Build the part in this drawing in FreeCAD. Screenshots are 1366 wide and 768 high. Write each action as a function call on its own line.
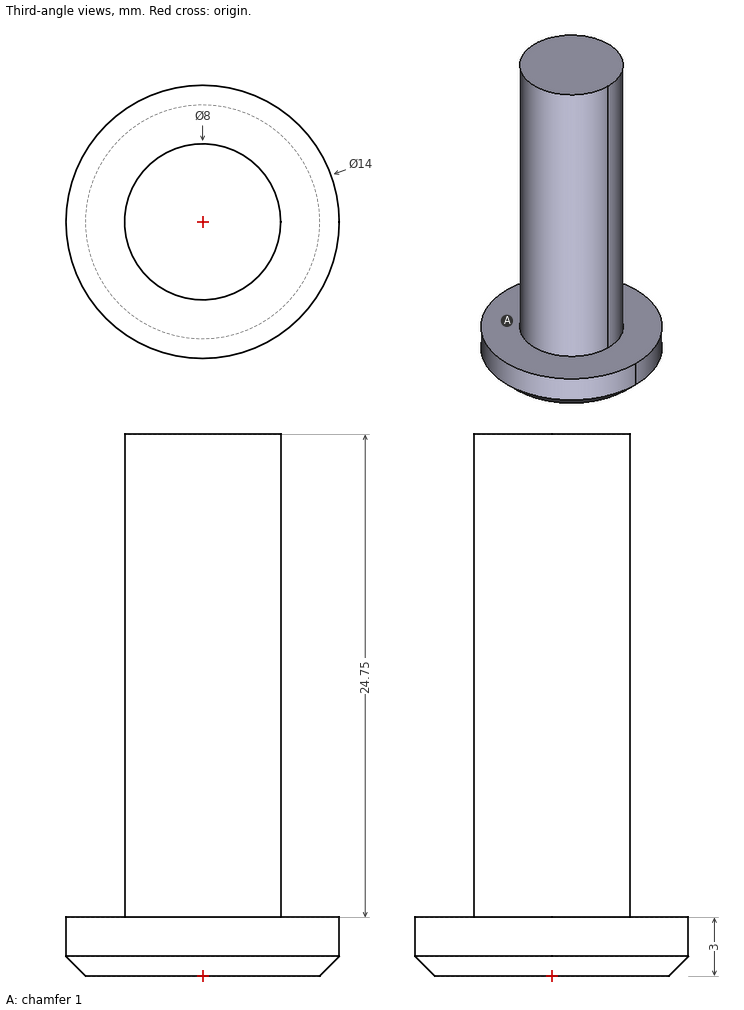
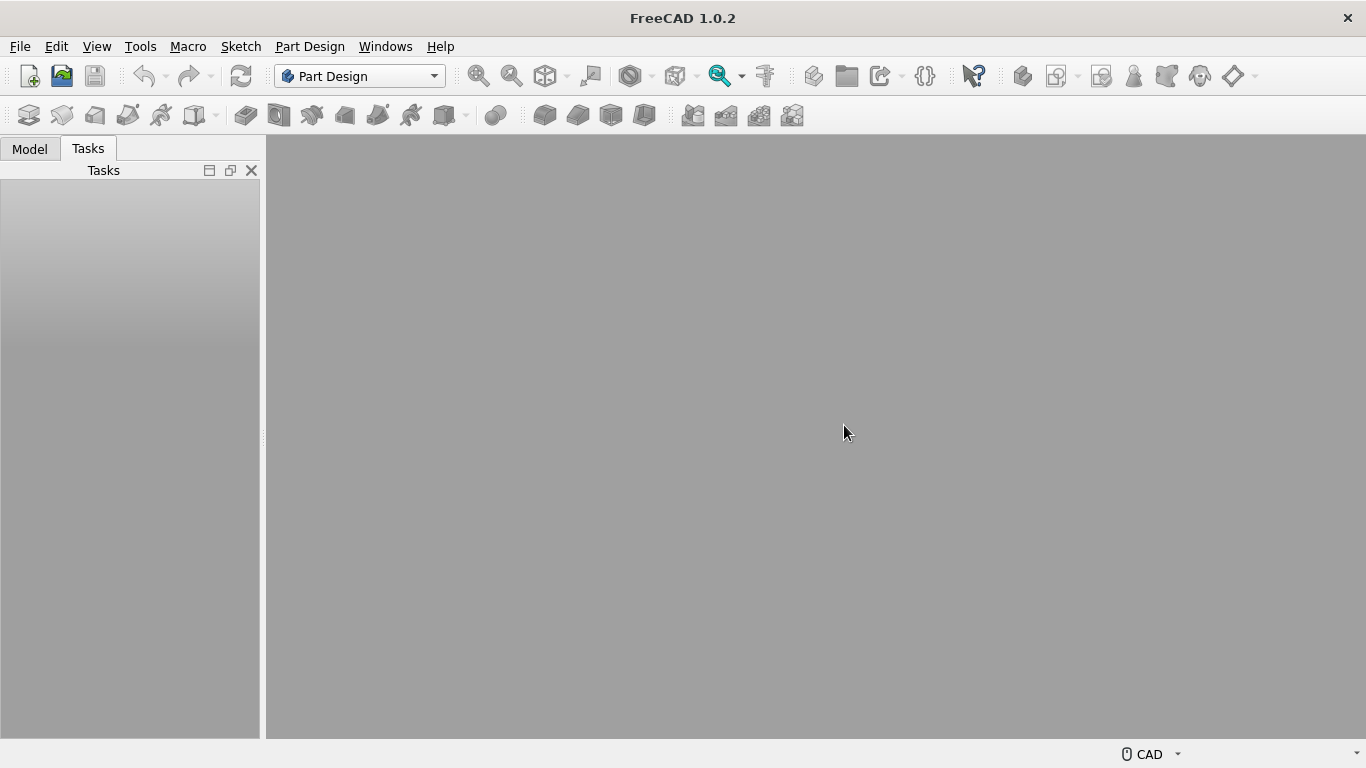
click(29, 76)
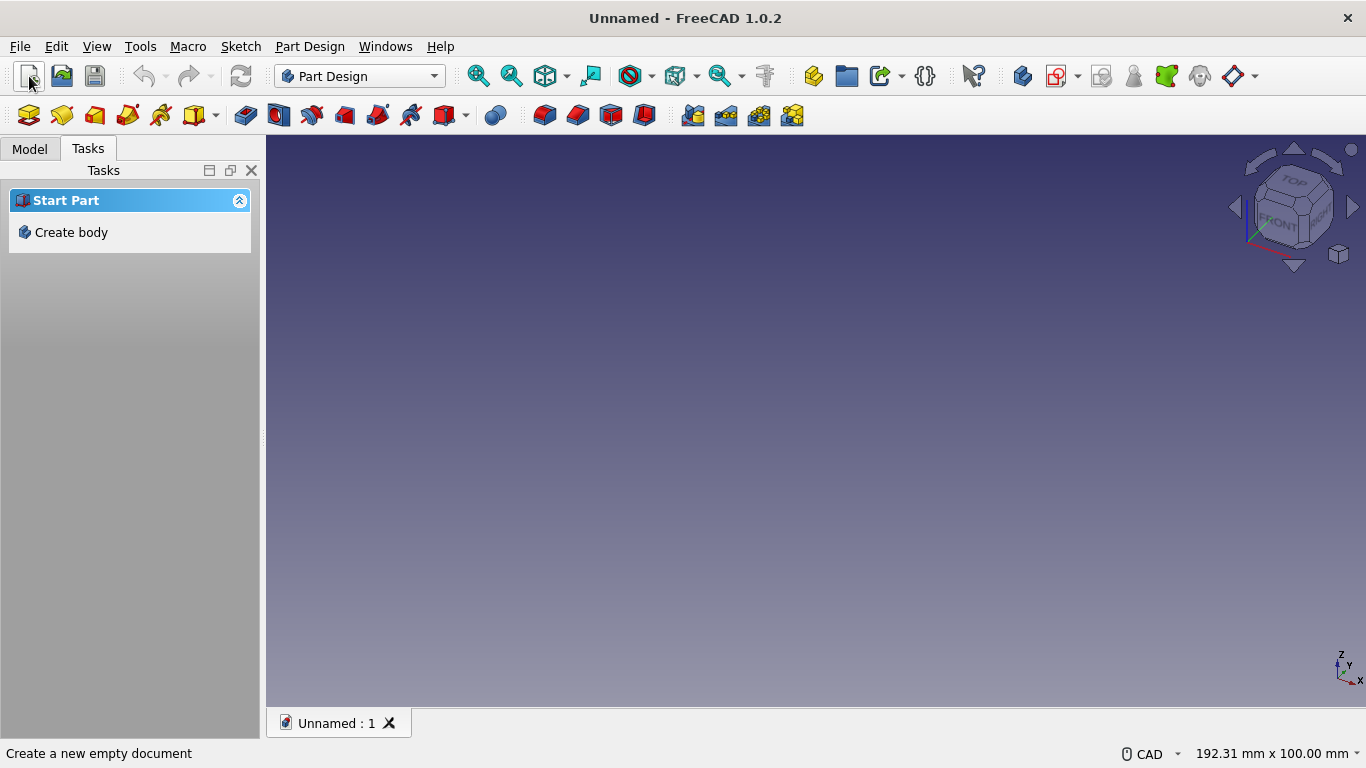
click(1056, 76)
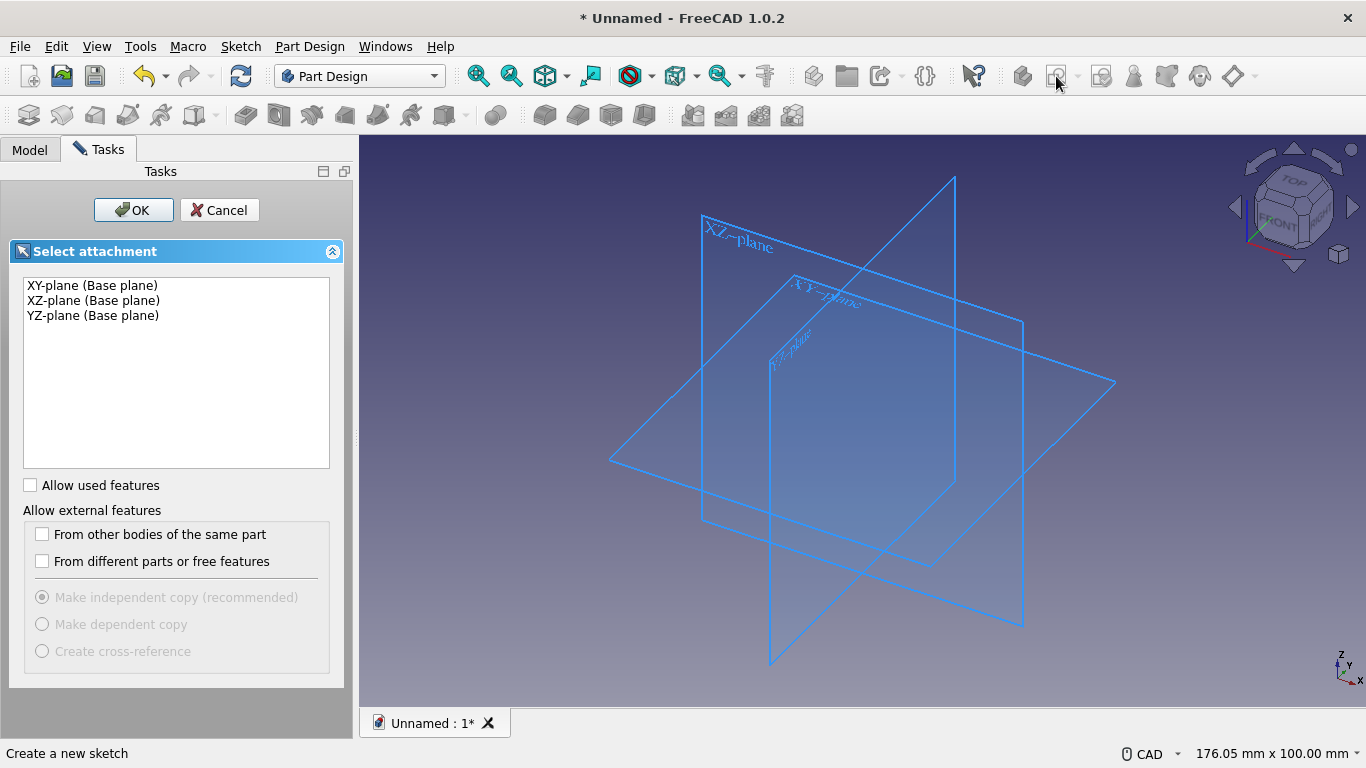
click(84, 286)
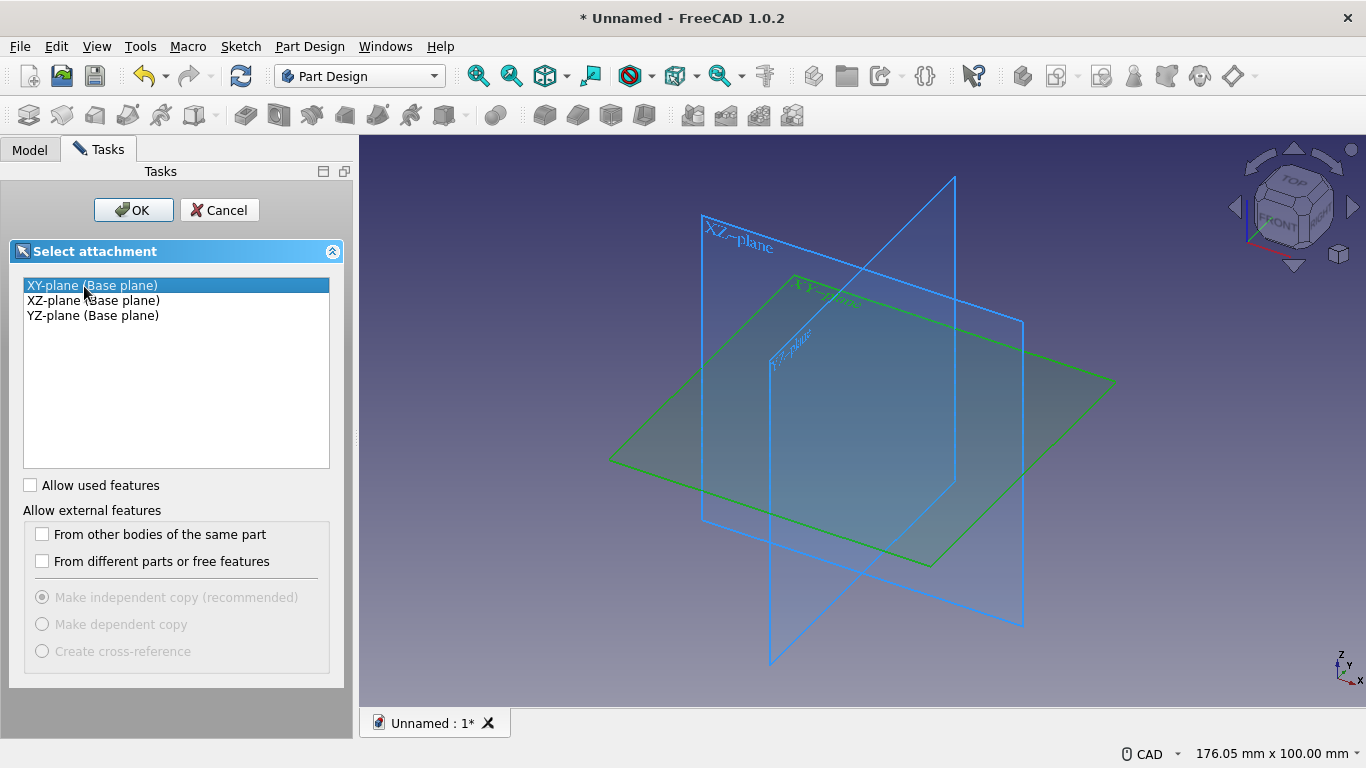
click(134, 210)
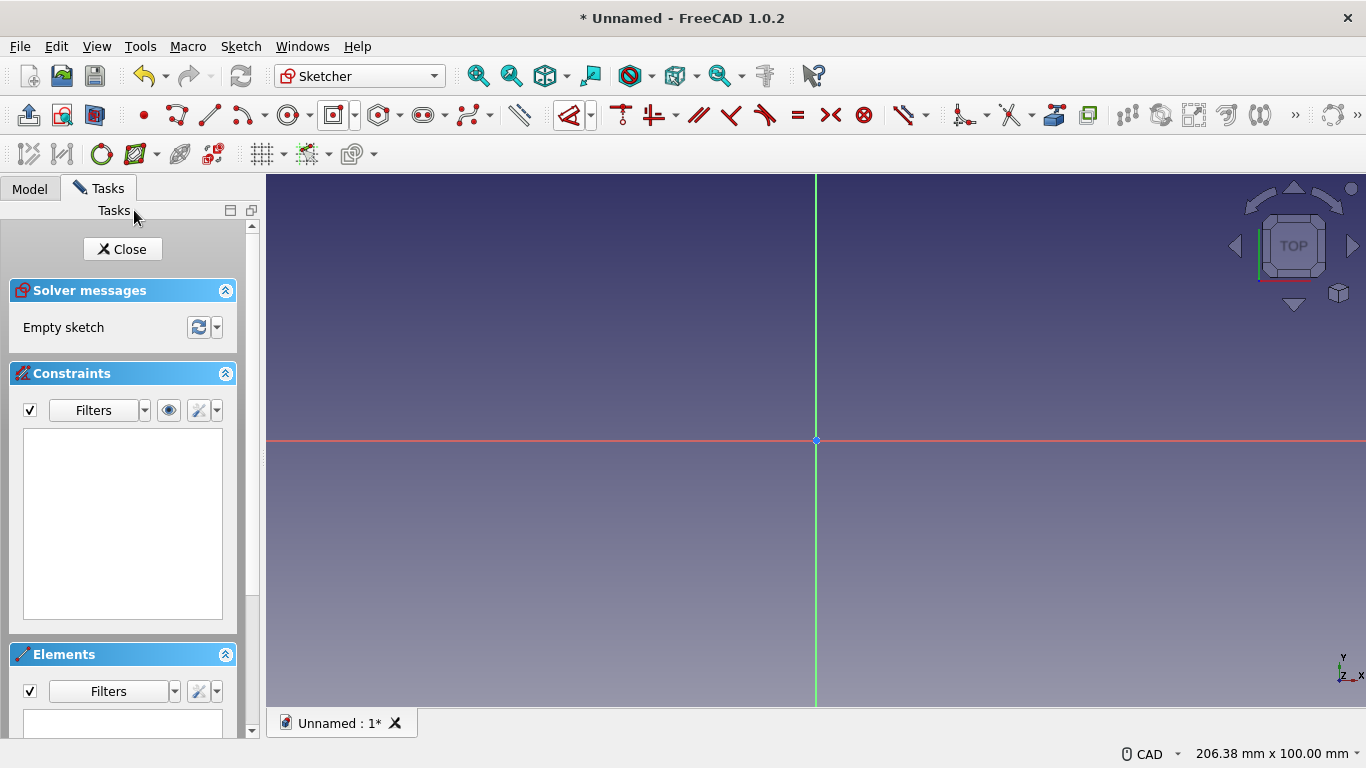
scroll(833, 440, up, 8)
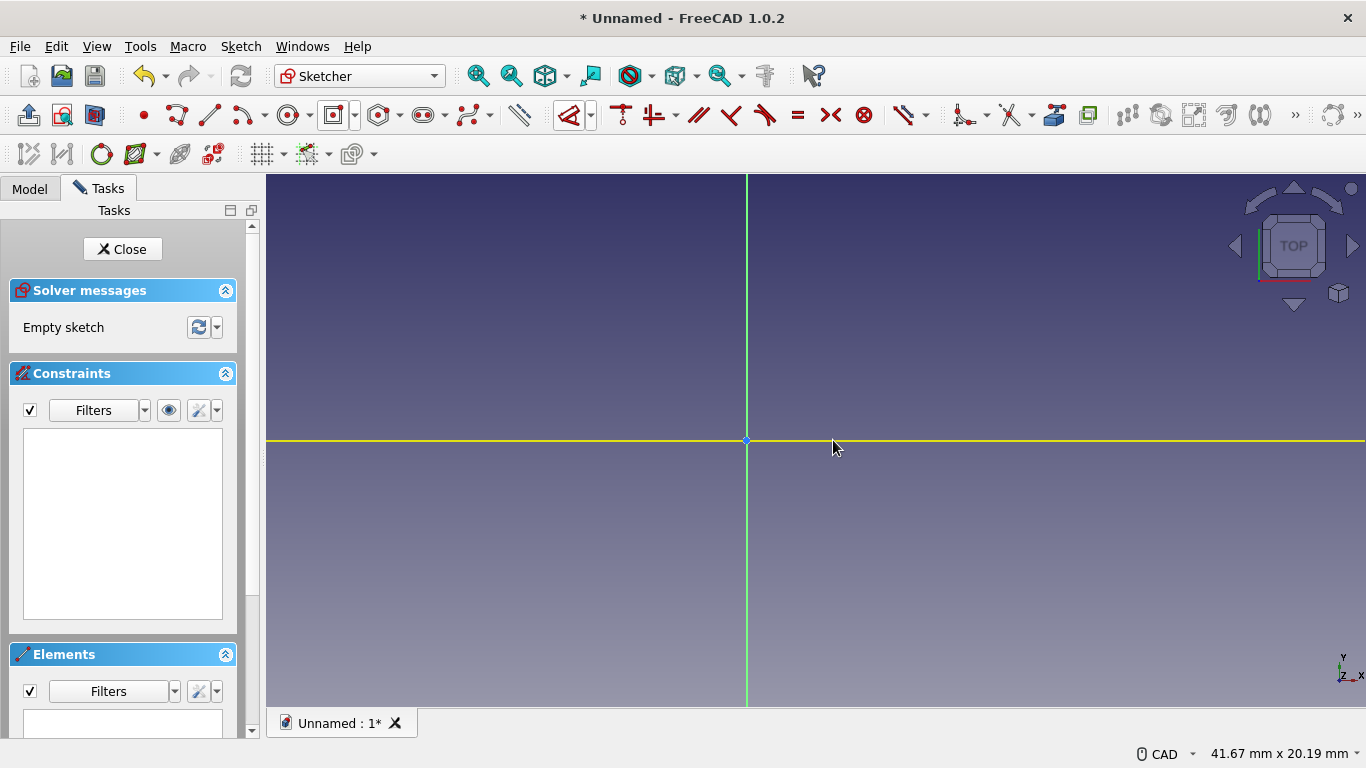
click(288, 116)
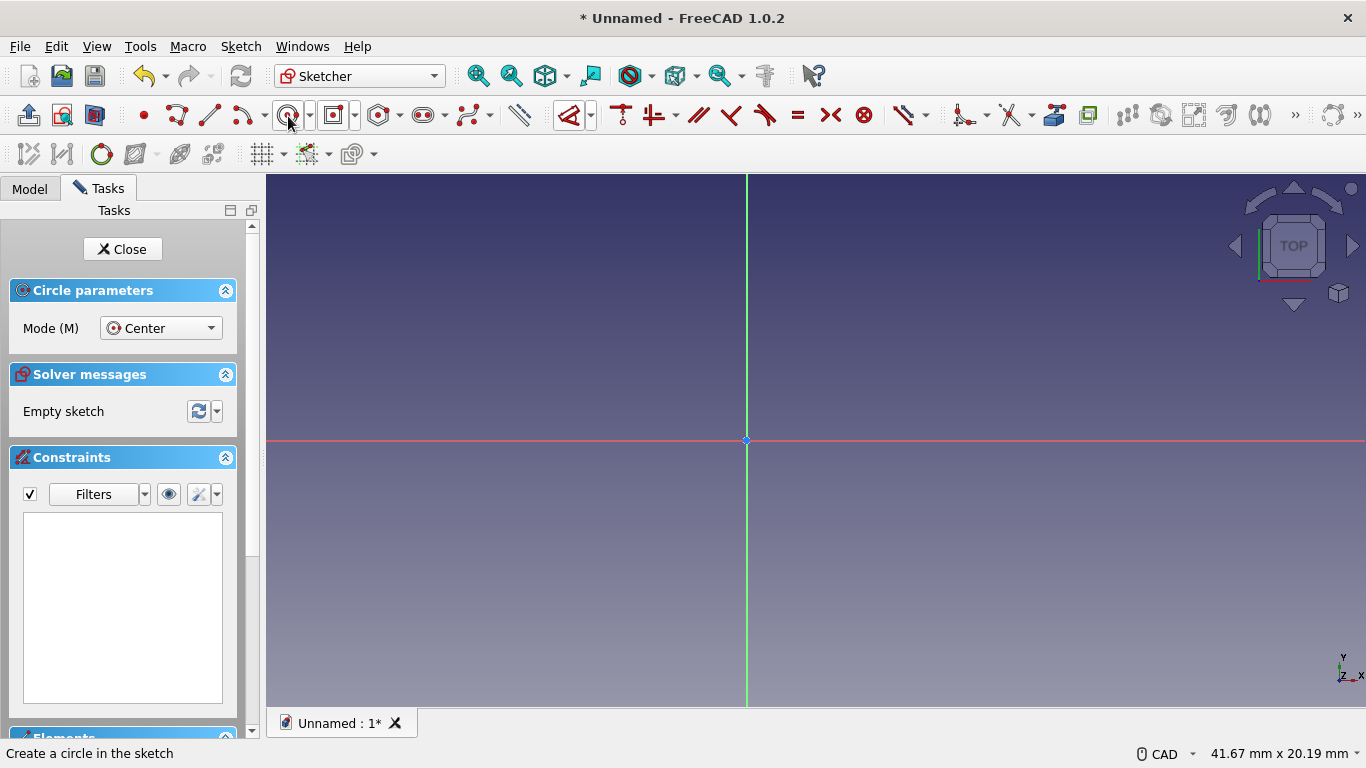
click(747, 440)
move(877, 310)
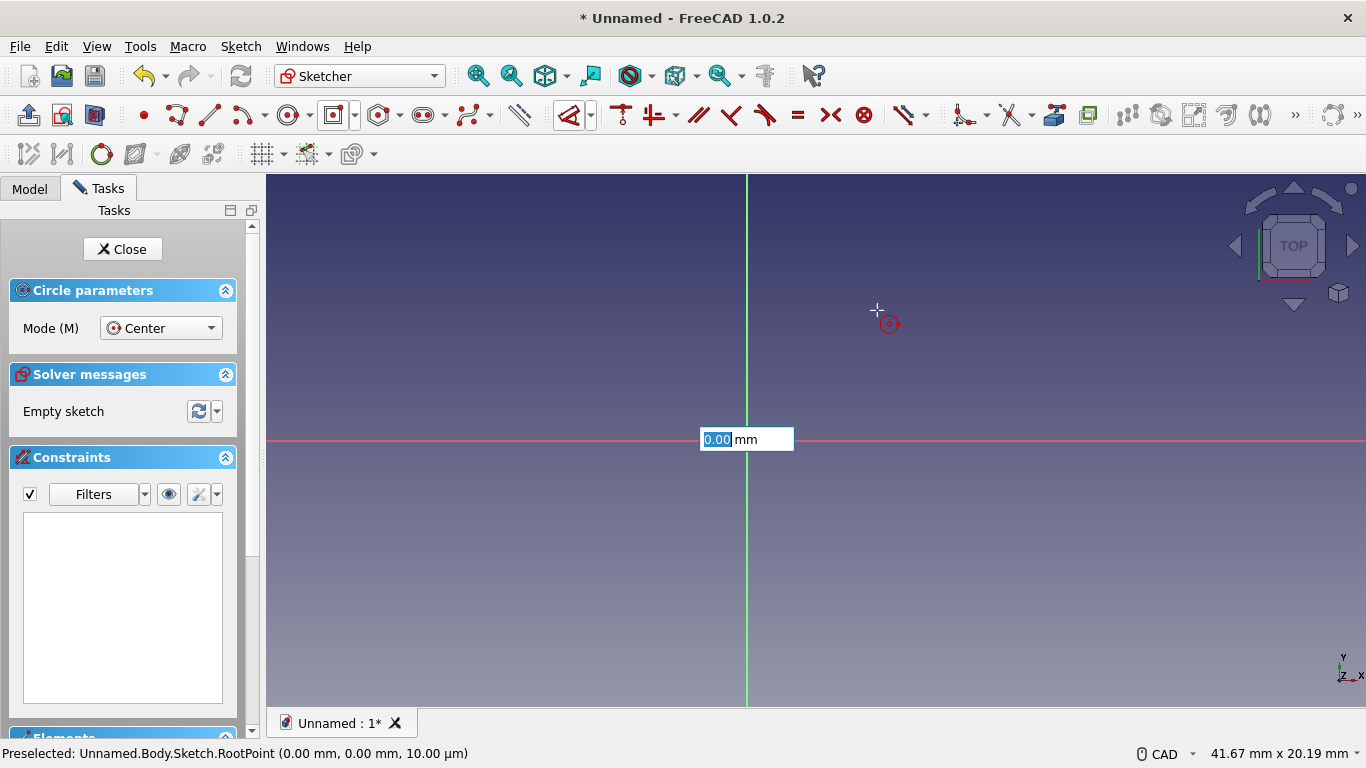
text(14)
key(Return)
key(Escape)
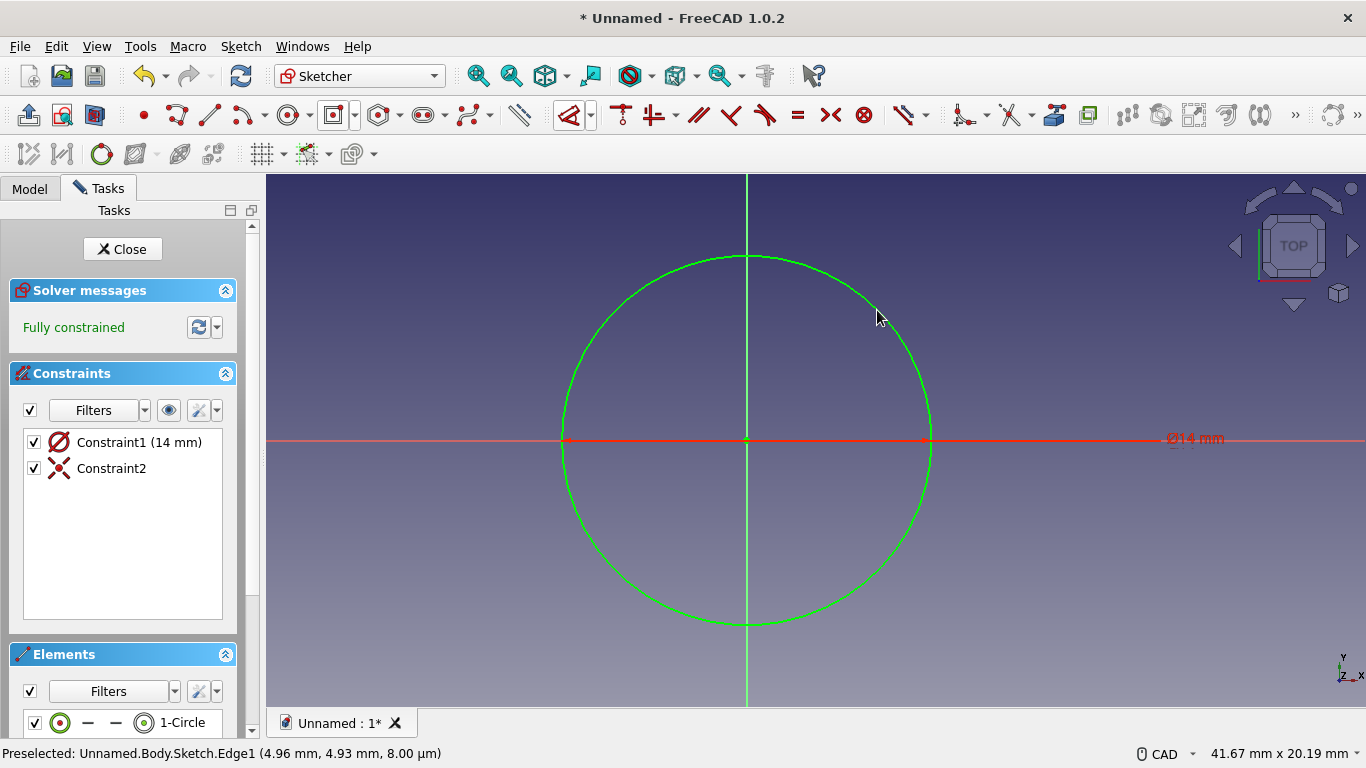
click(123, 249)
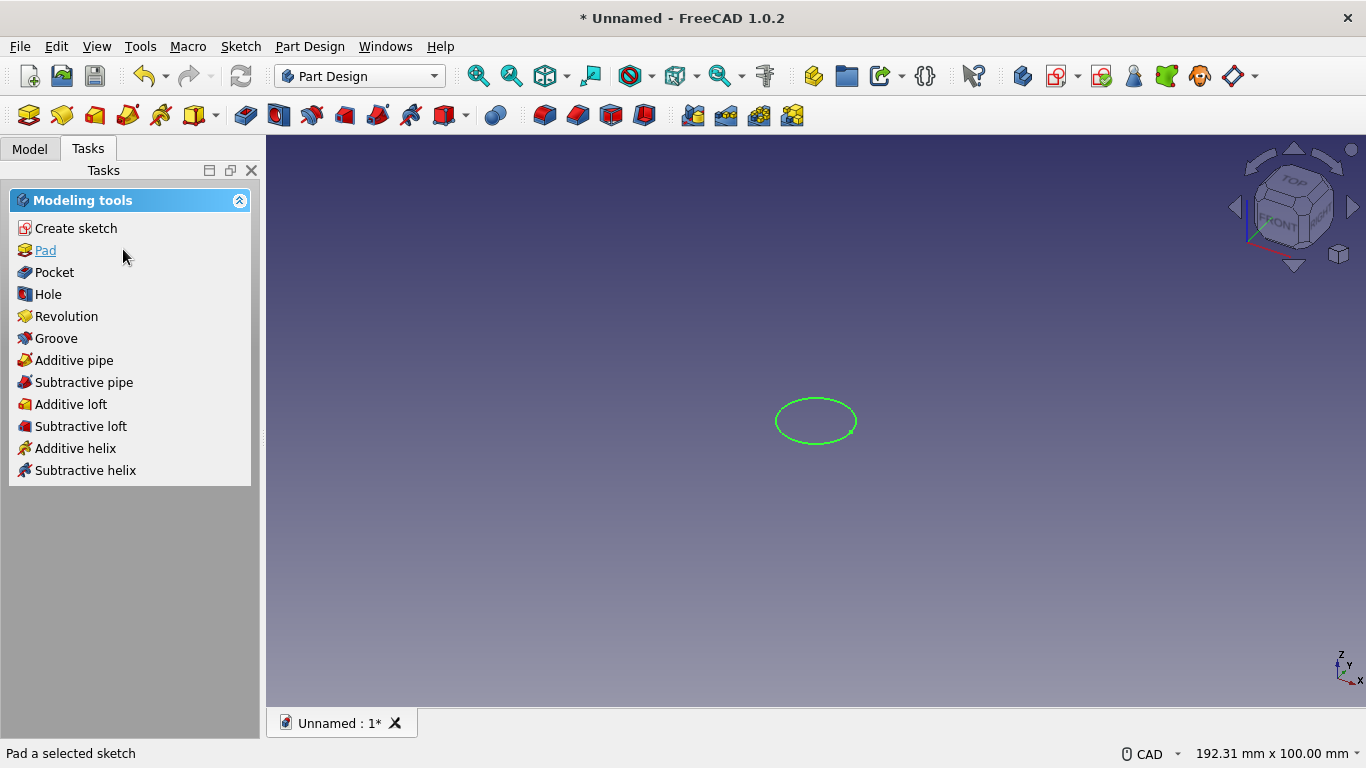
click(29, 116)